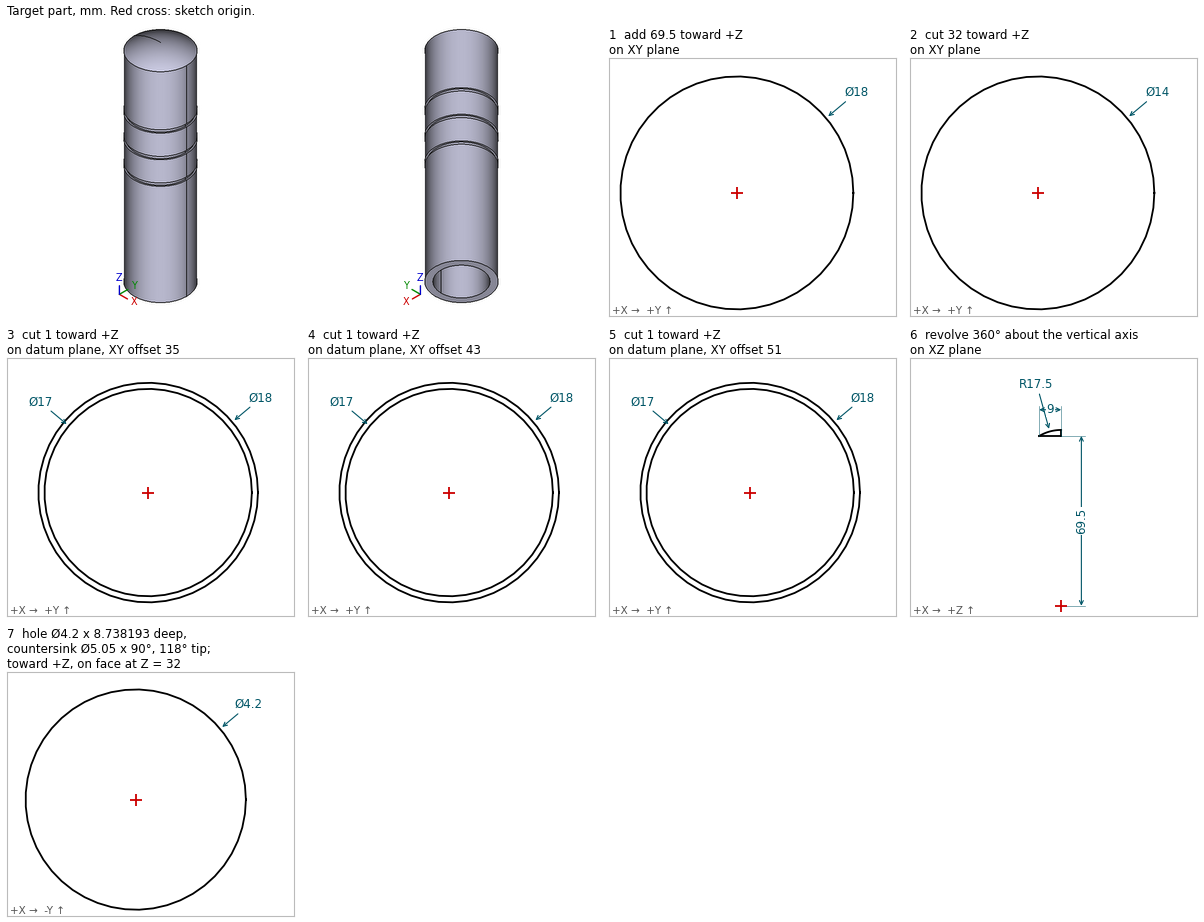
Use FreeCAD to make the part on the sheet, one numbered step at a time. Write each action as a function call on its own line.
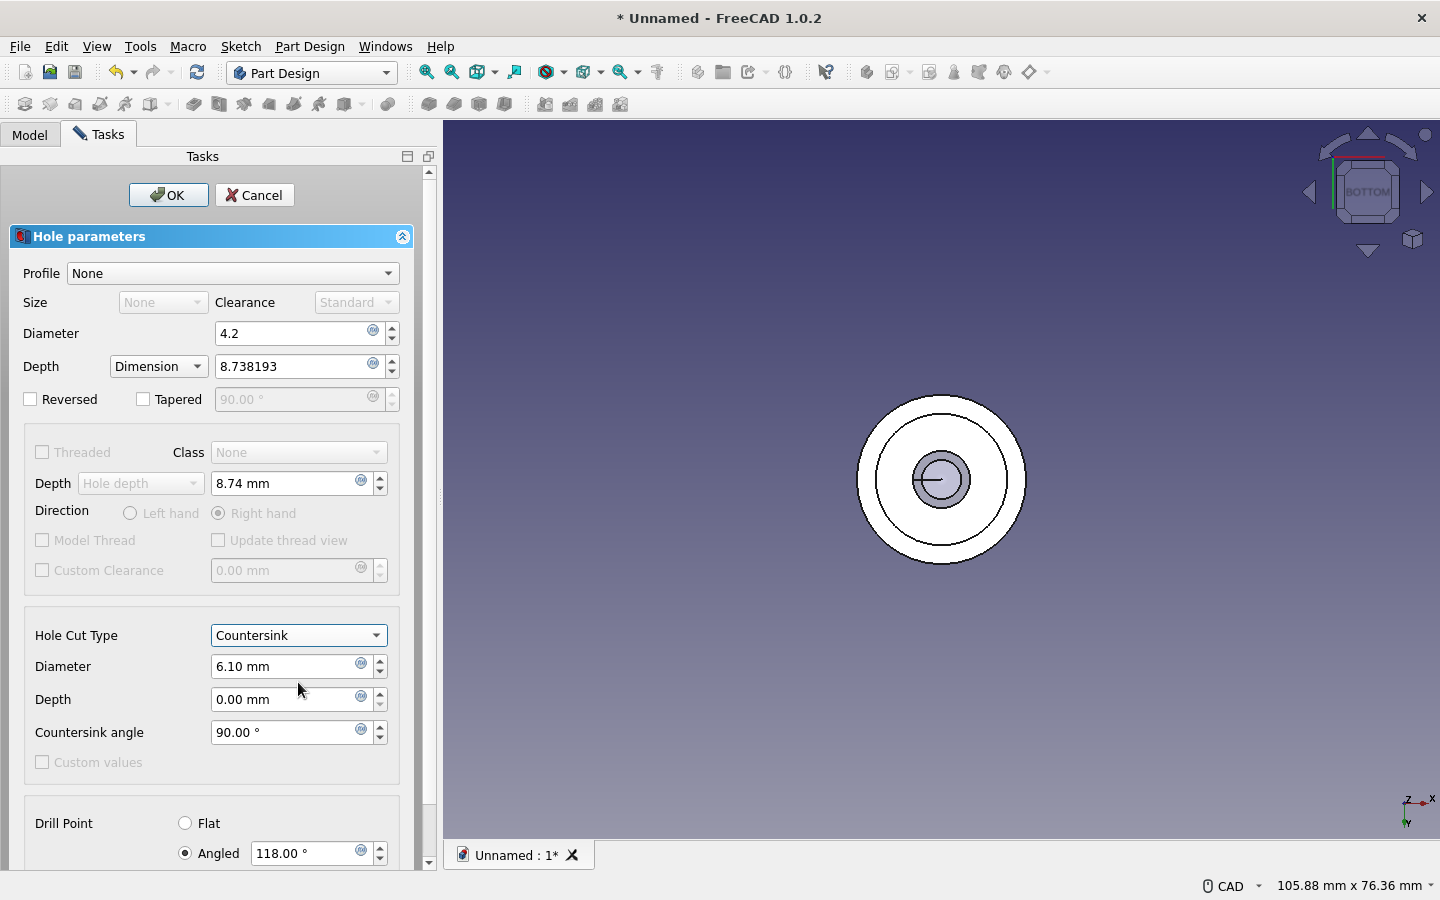
triple_click(292, 666)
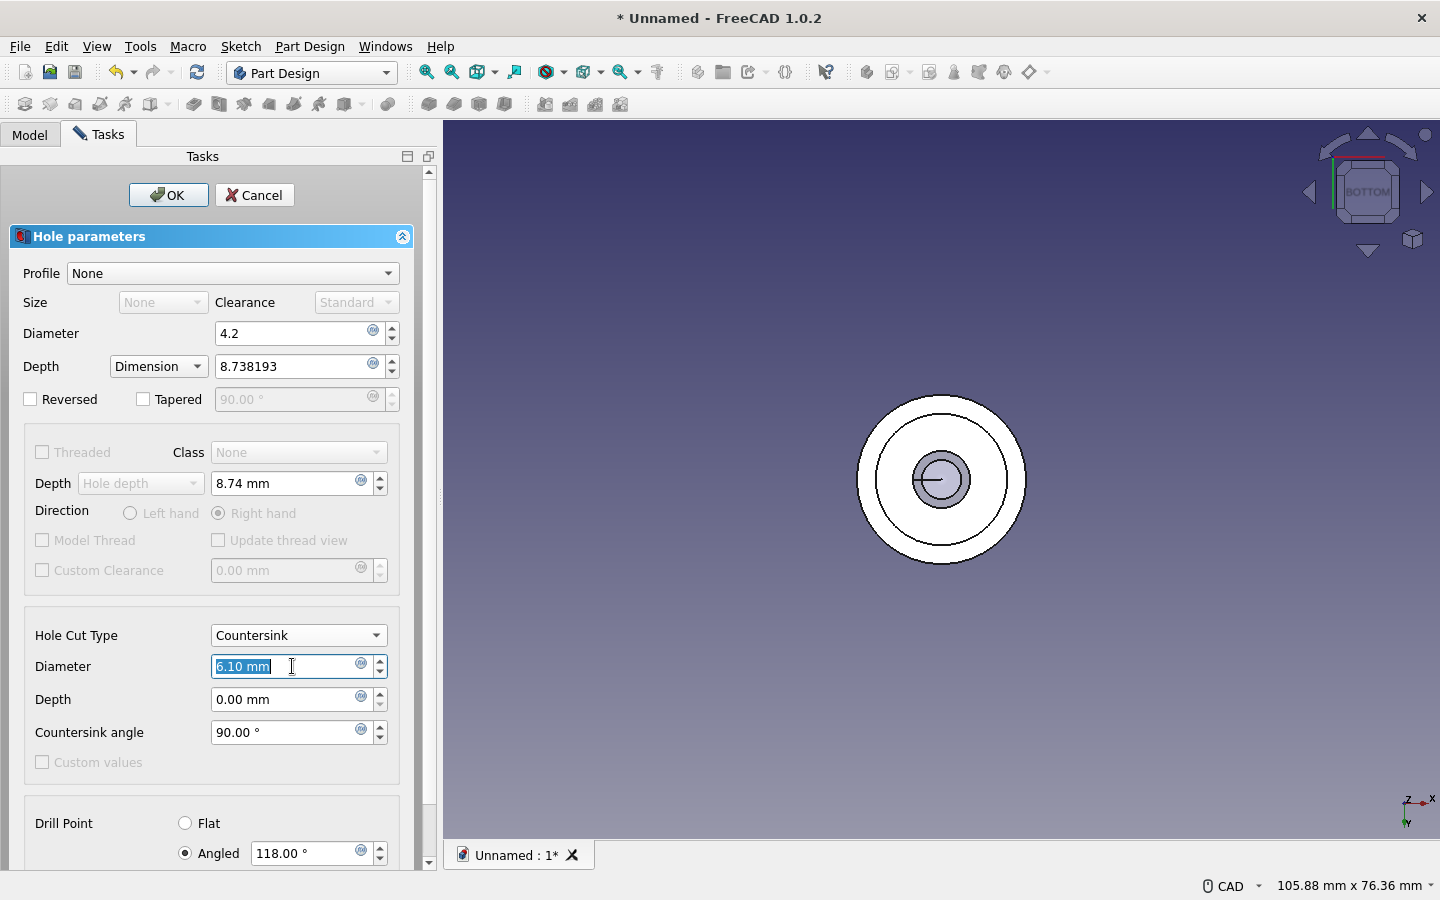
text(5.05)
key(Tab)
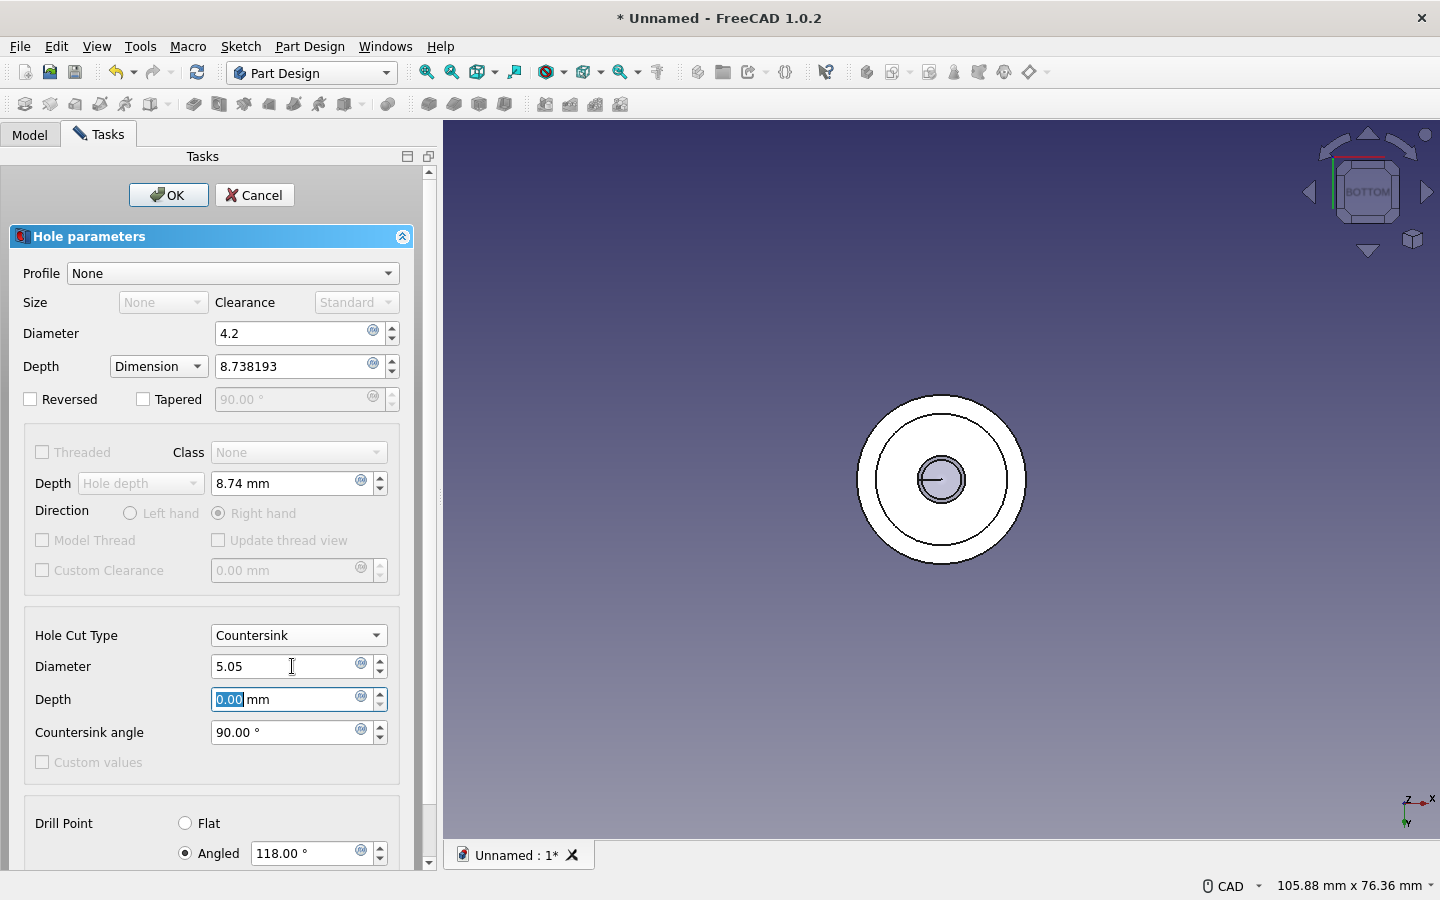
click(169, 195)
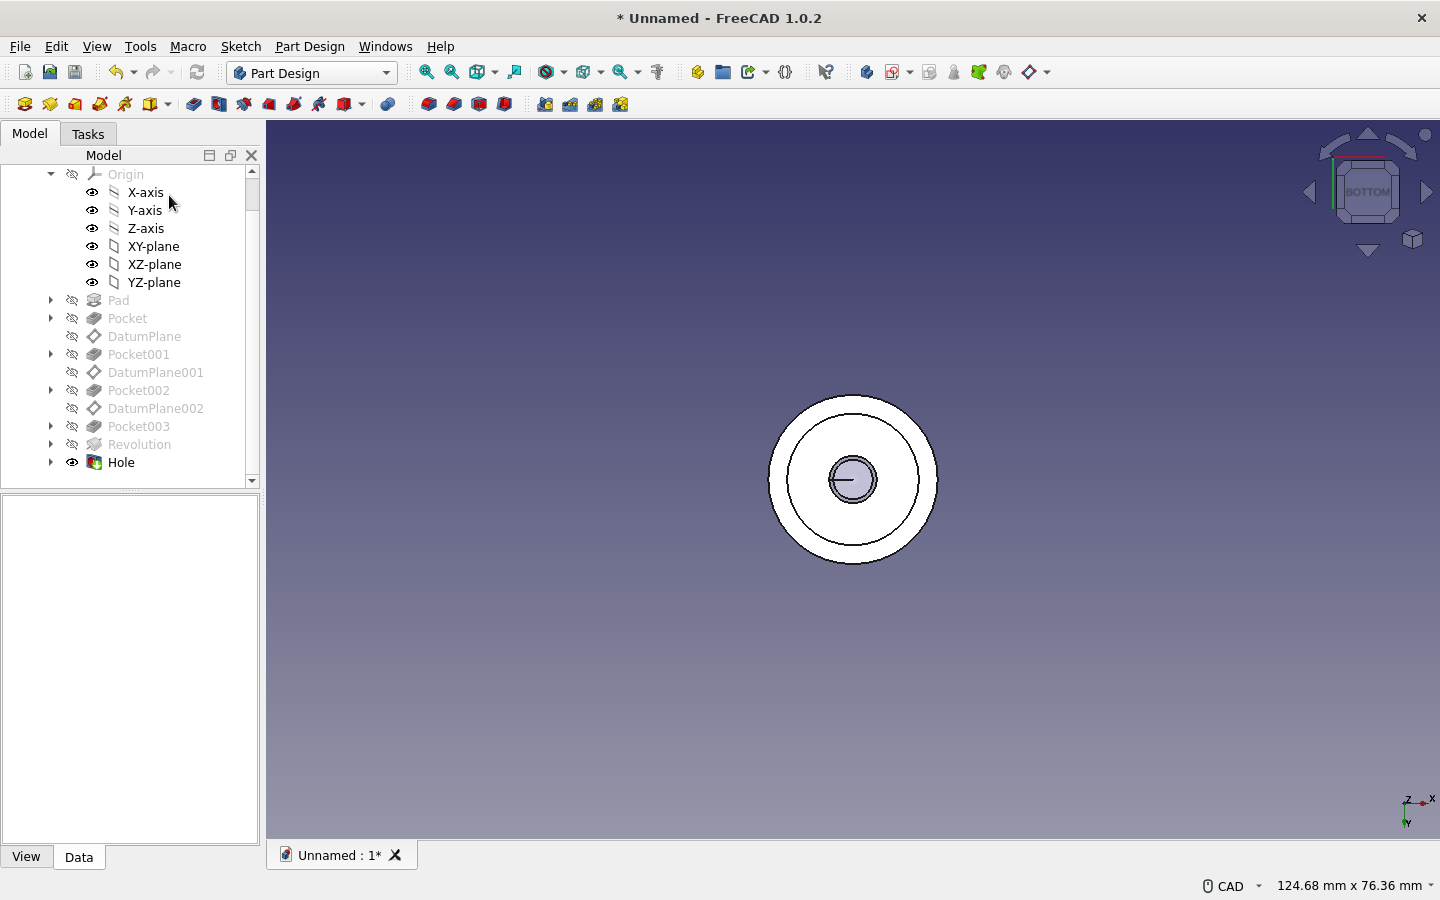
key(0)